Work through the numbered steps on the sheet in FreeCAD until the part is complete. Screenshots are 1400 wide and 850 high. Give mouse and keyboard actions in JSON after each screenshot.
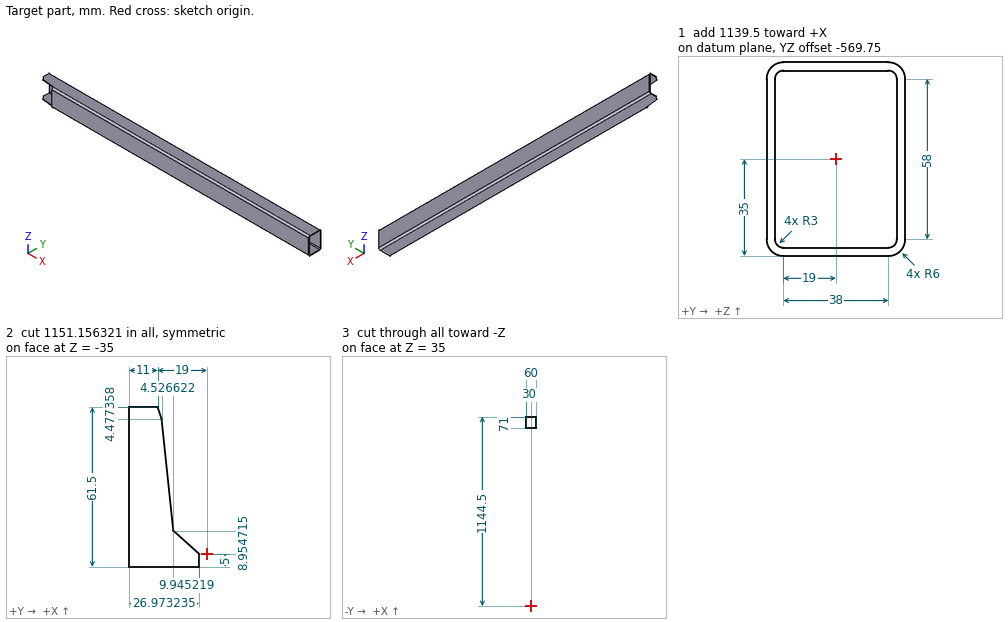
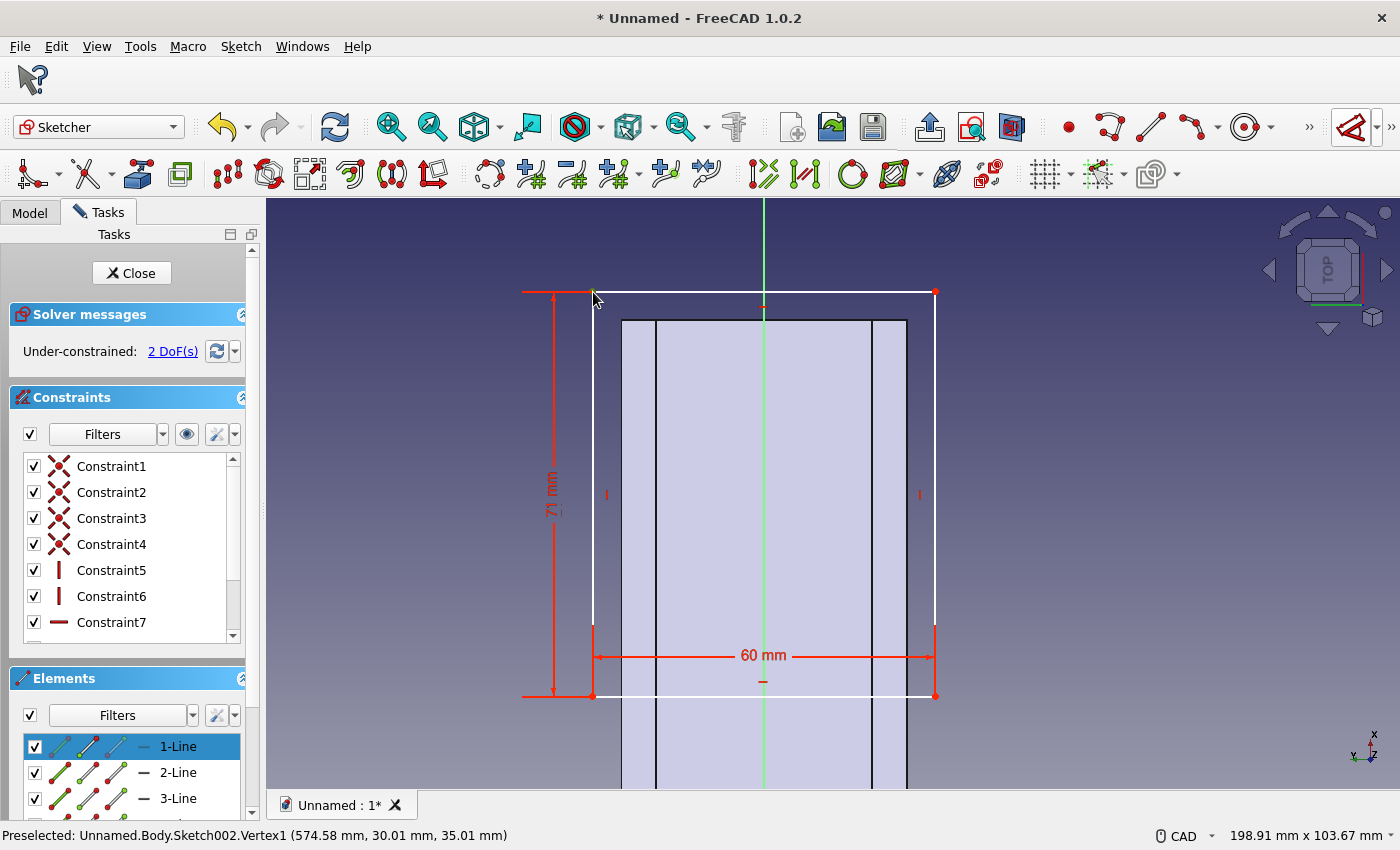
{"action": "key", "text": "l"}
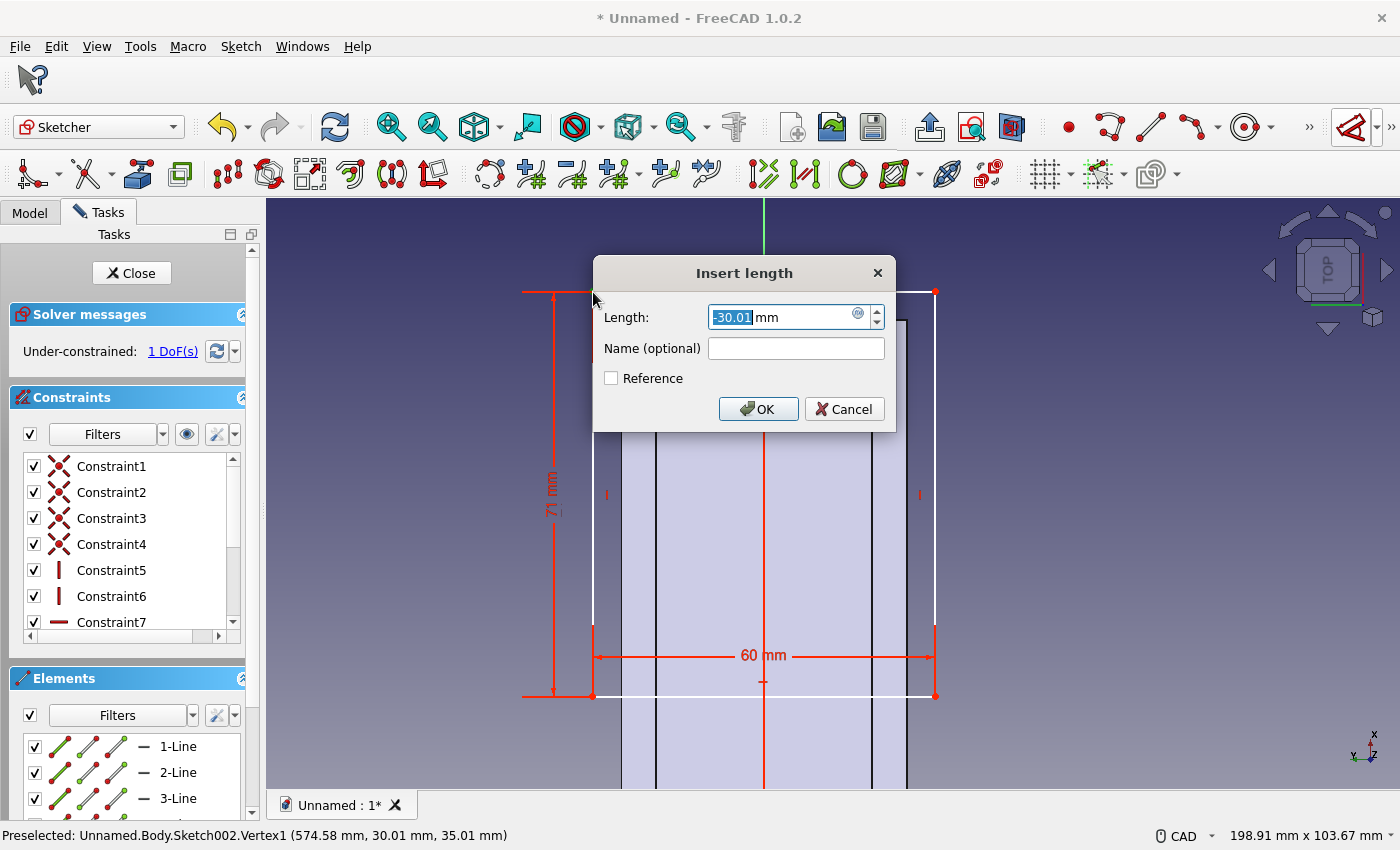
{"action": "type", "text": "-30"}
{"action": "key", "text": "Return"}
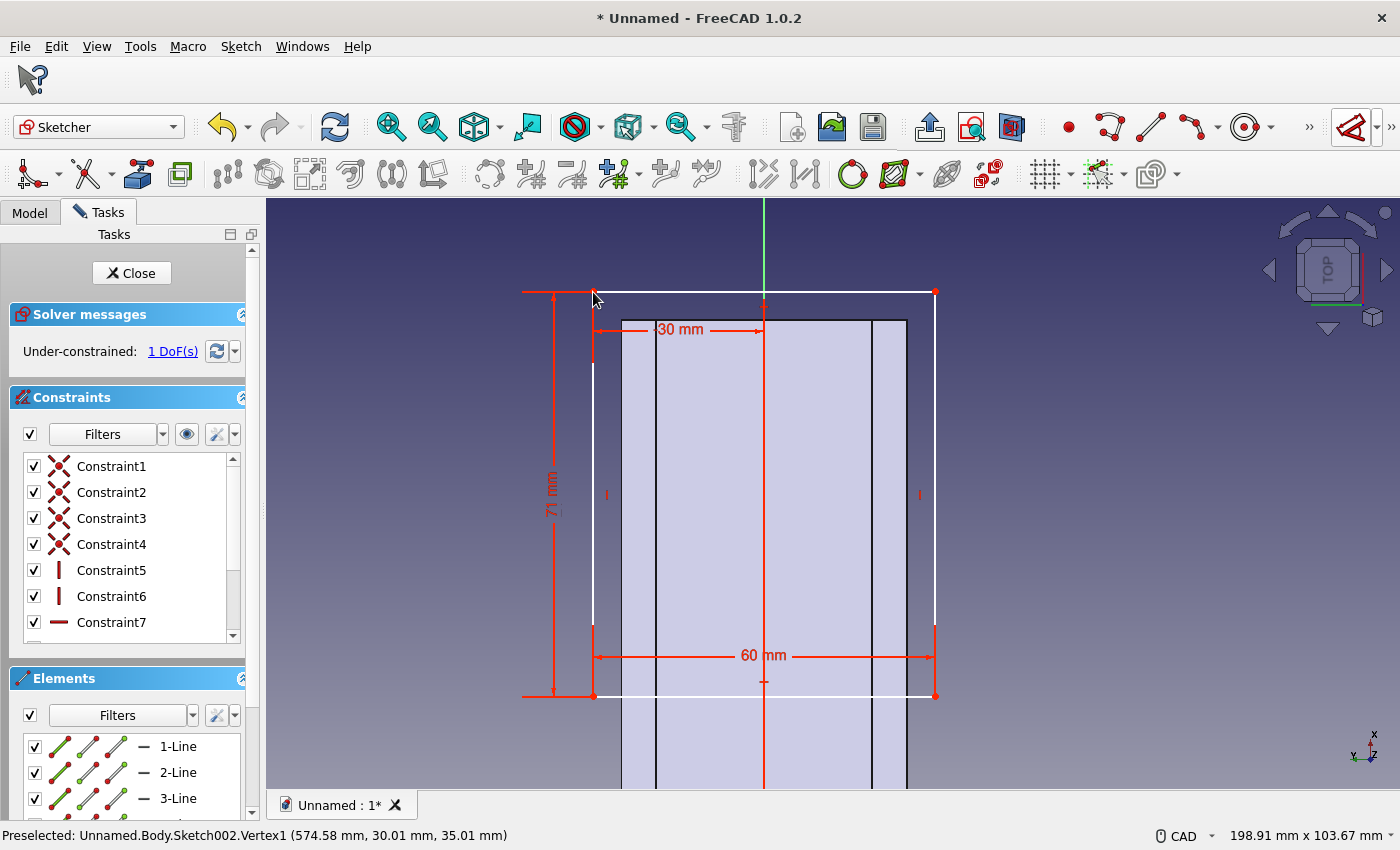
{"action": "left_click", "coordinate": [593, 292]}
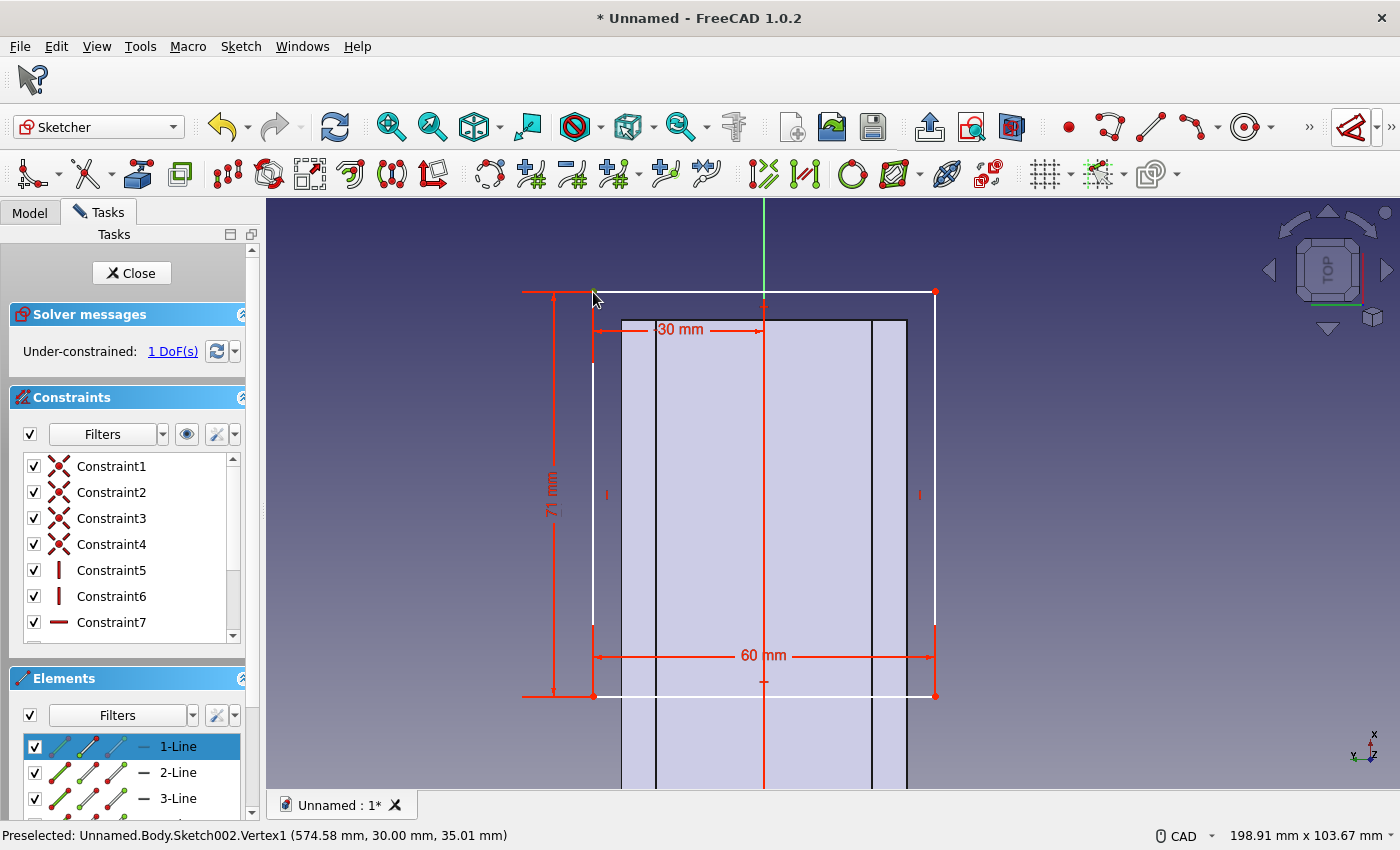
{"action": "left_click", "coordinate": [1376, 128]}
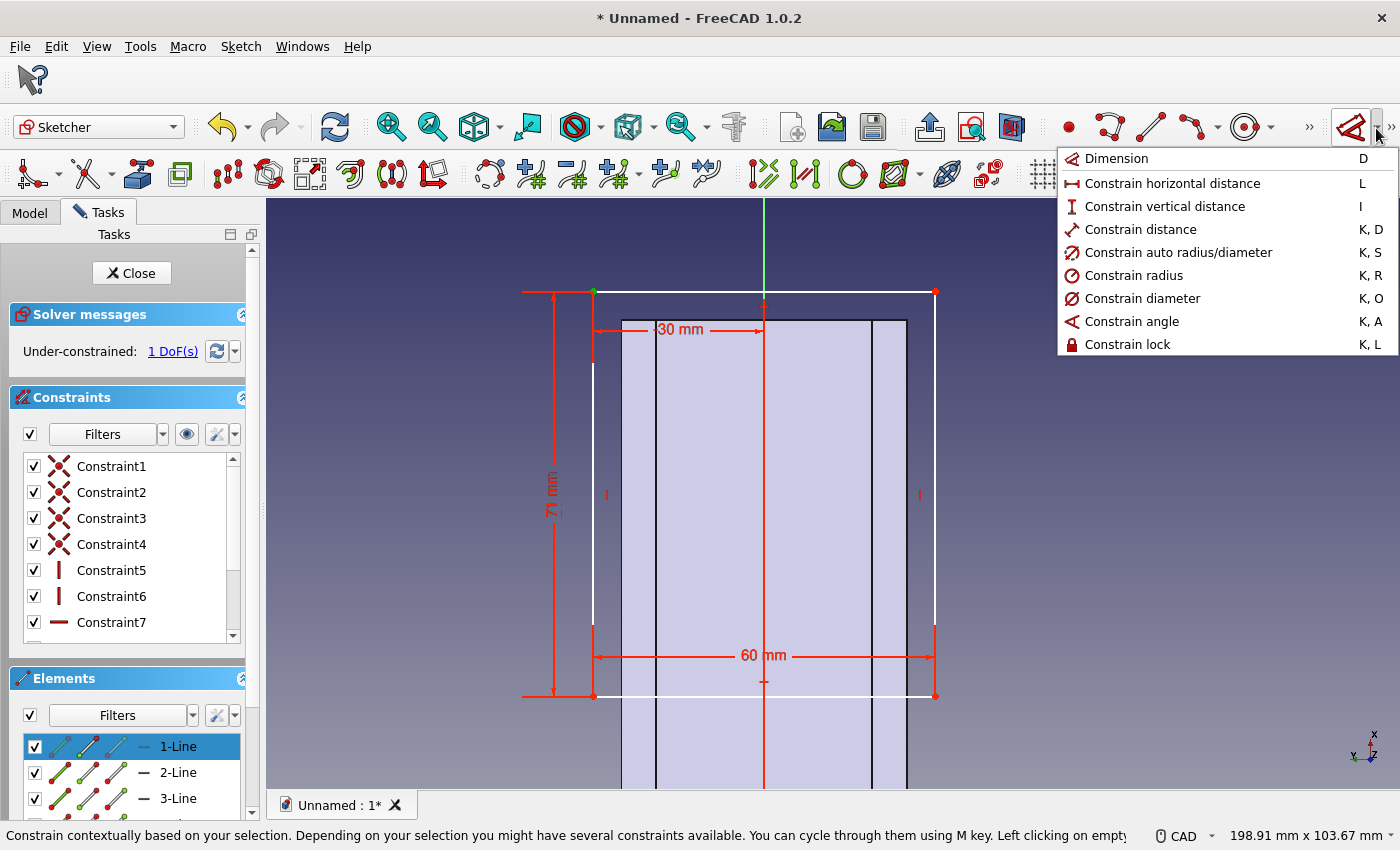
{"action": "left_click", "coordinate": [1228, 206]}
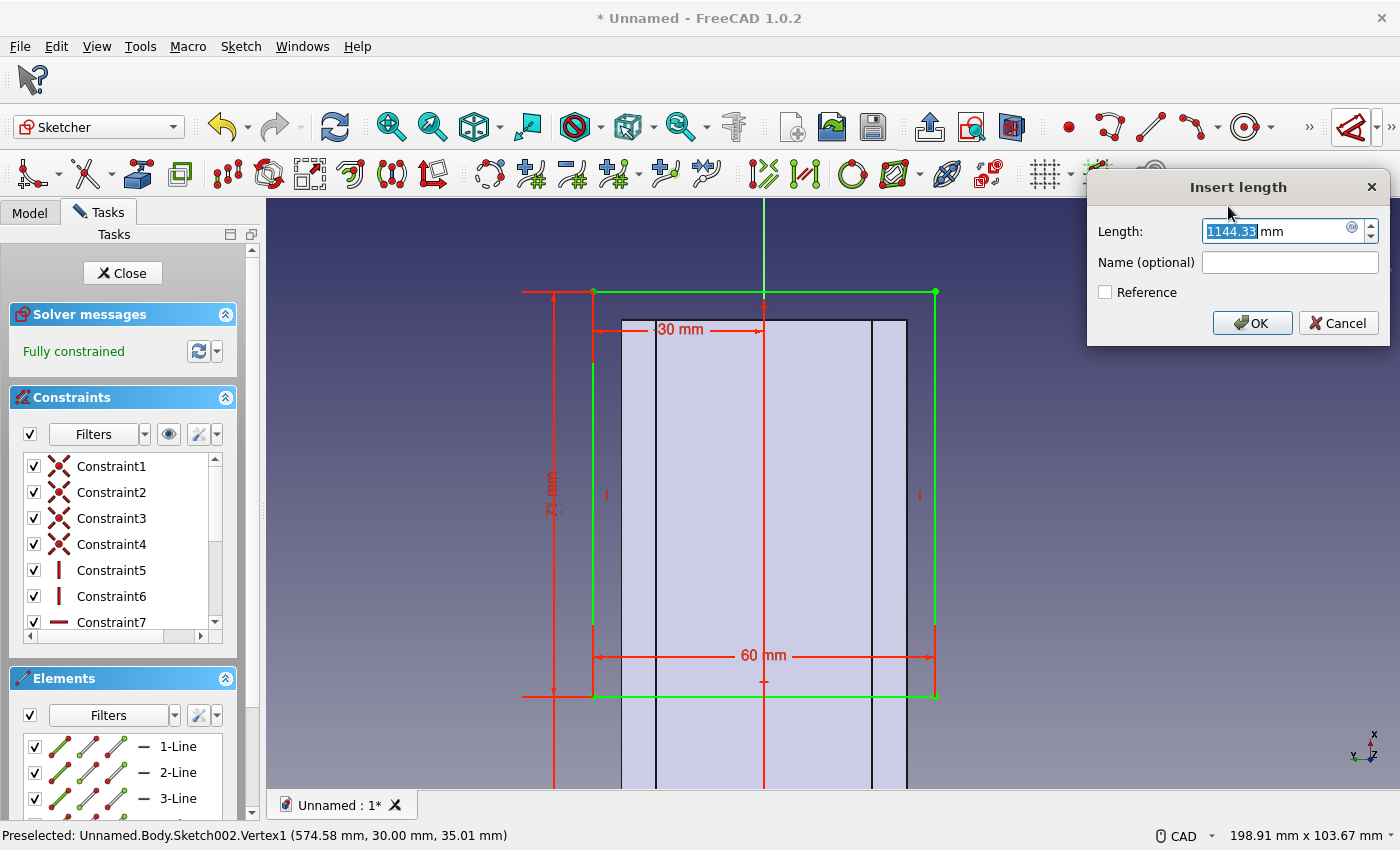
{"action": "type", "text": "1144.5"}
{"action": "key", "text": "Return"}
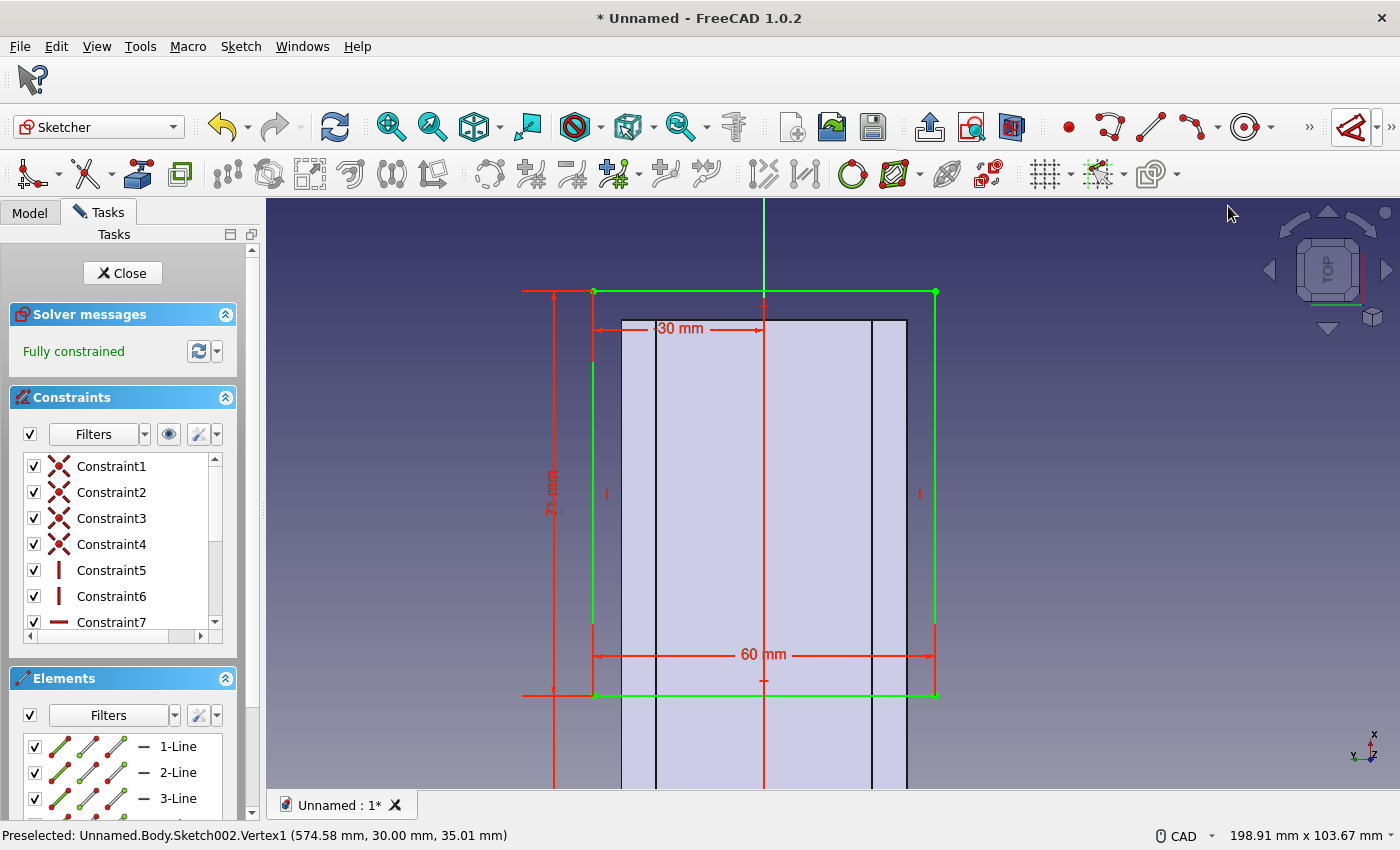
{"action": "left_click", "coordinate": [123, 273]}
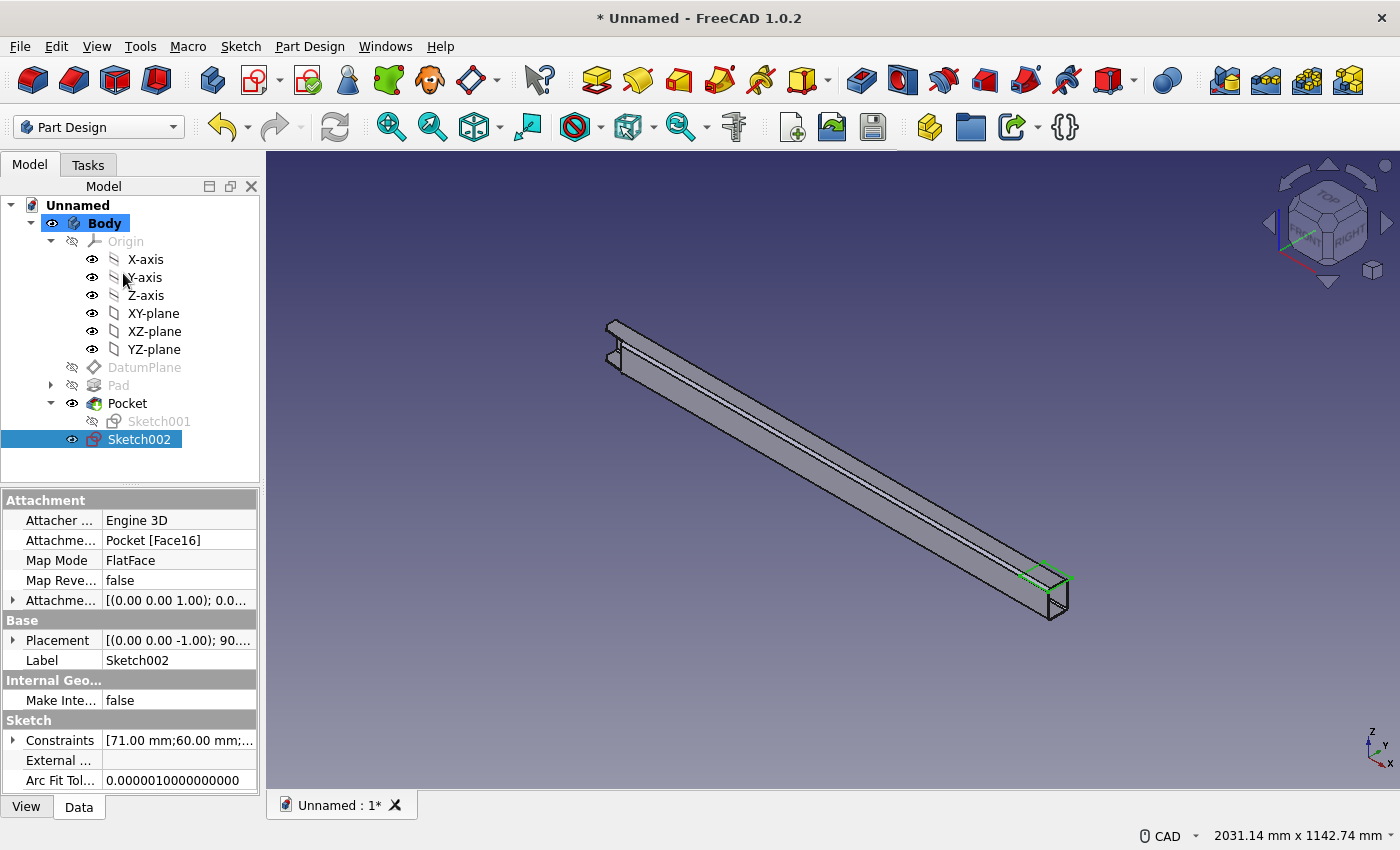
{"action": "left_click", "coordinate": [862, 80]}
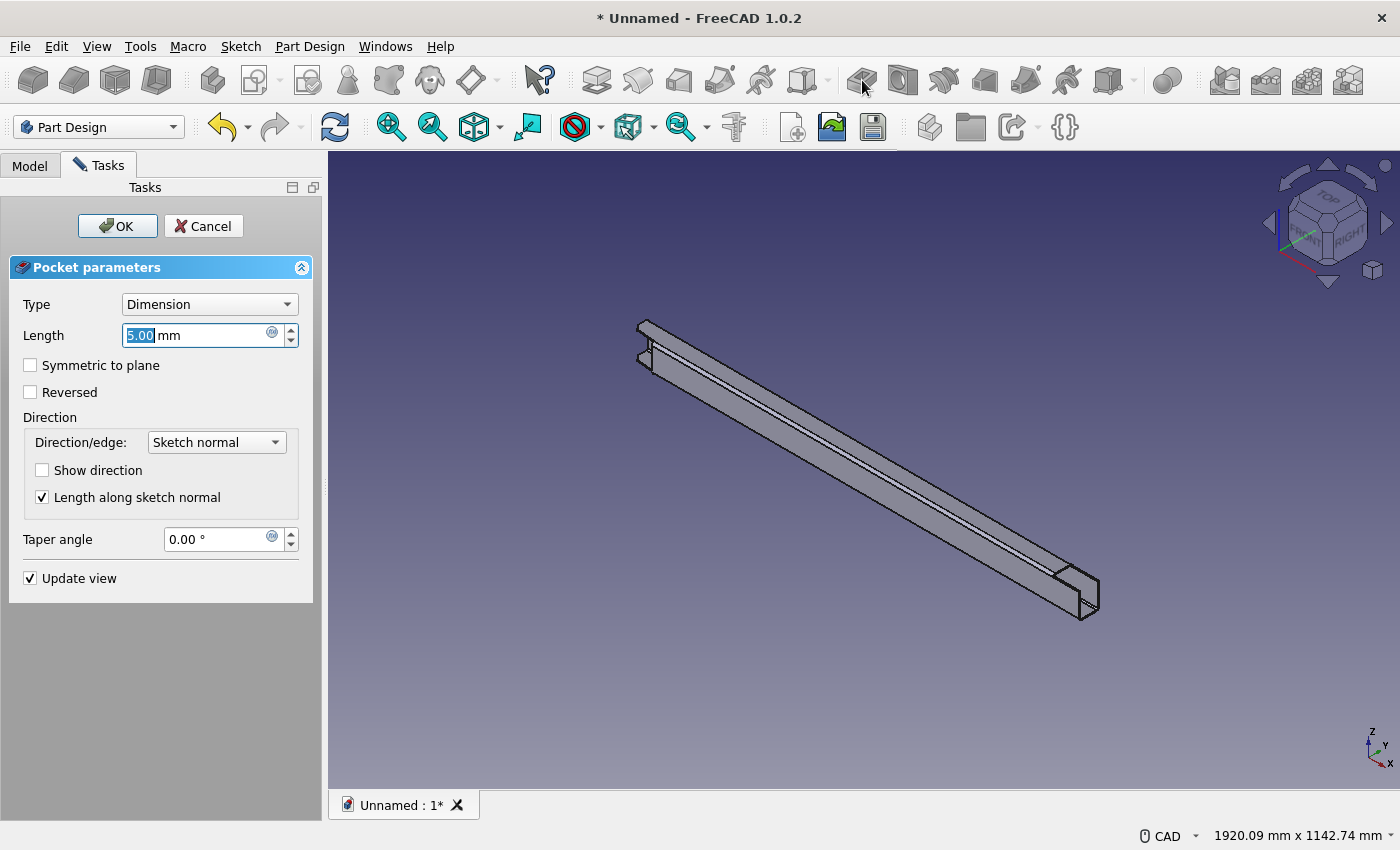
{"action": "left_click", "coordinate": [210, 304]}